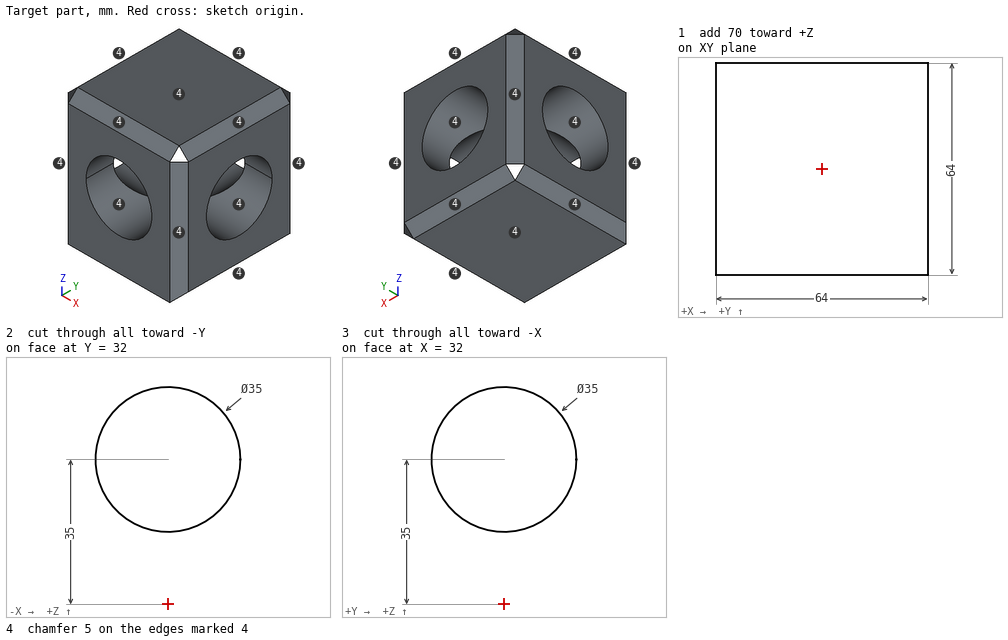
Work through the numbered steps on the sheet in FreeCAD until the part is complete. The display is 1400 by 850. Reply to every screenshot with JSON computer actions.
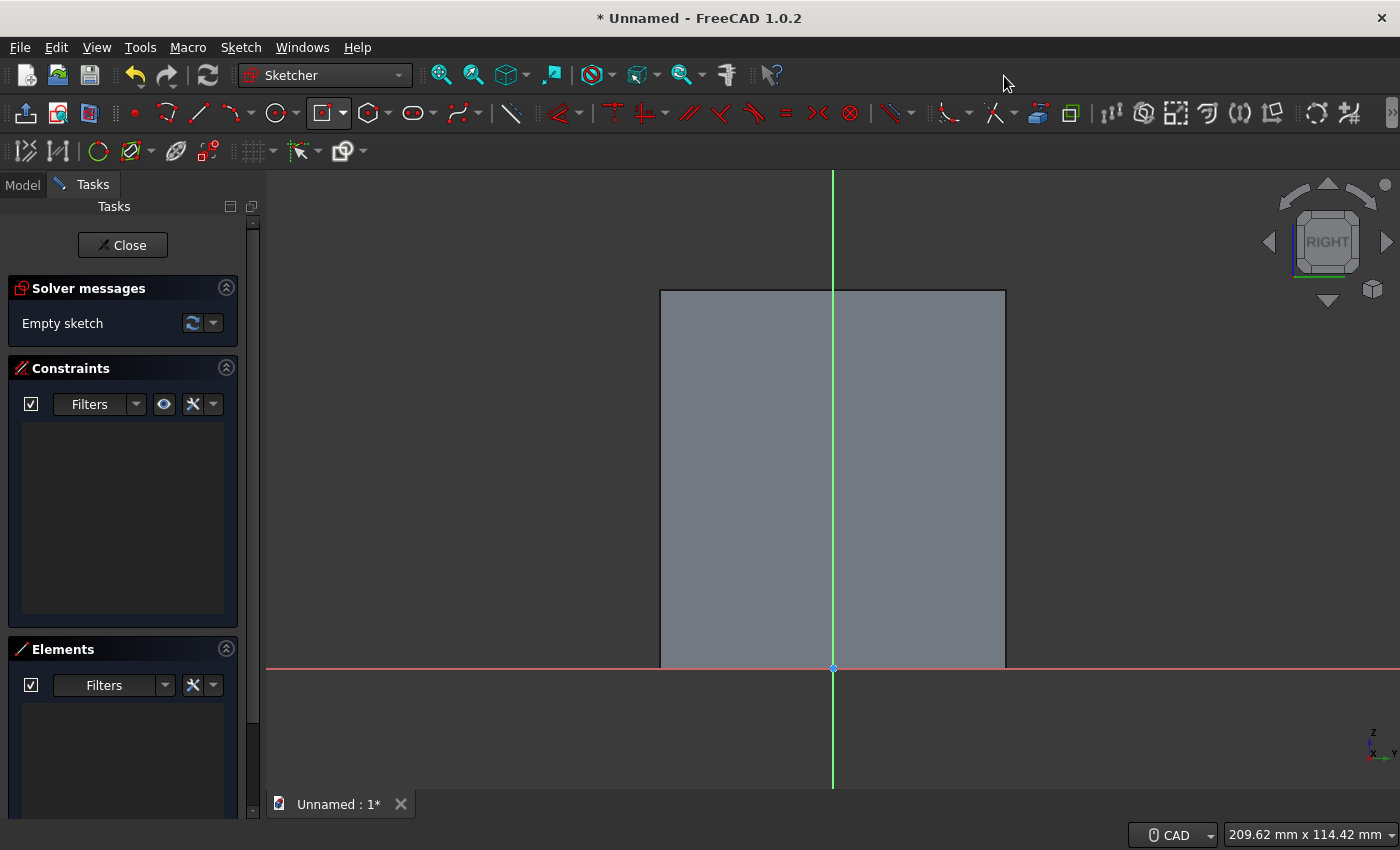
{"action": "scroll", "coordinate": [972, 623], "scroll_direction": "up", "scroll_amount": 2}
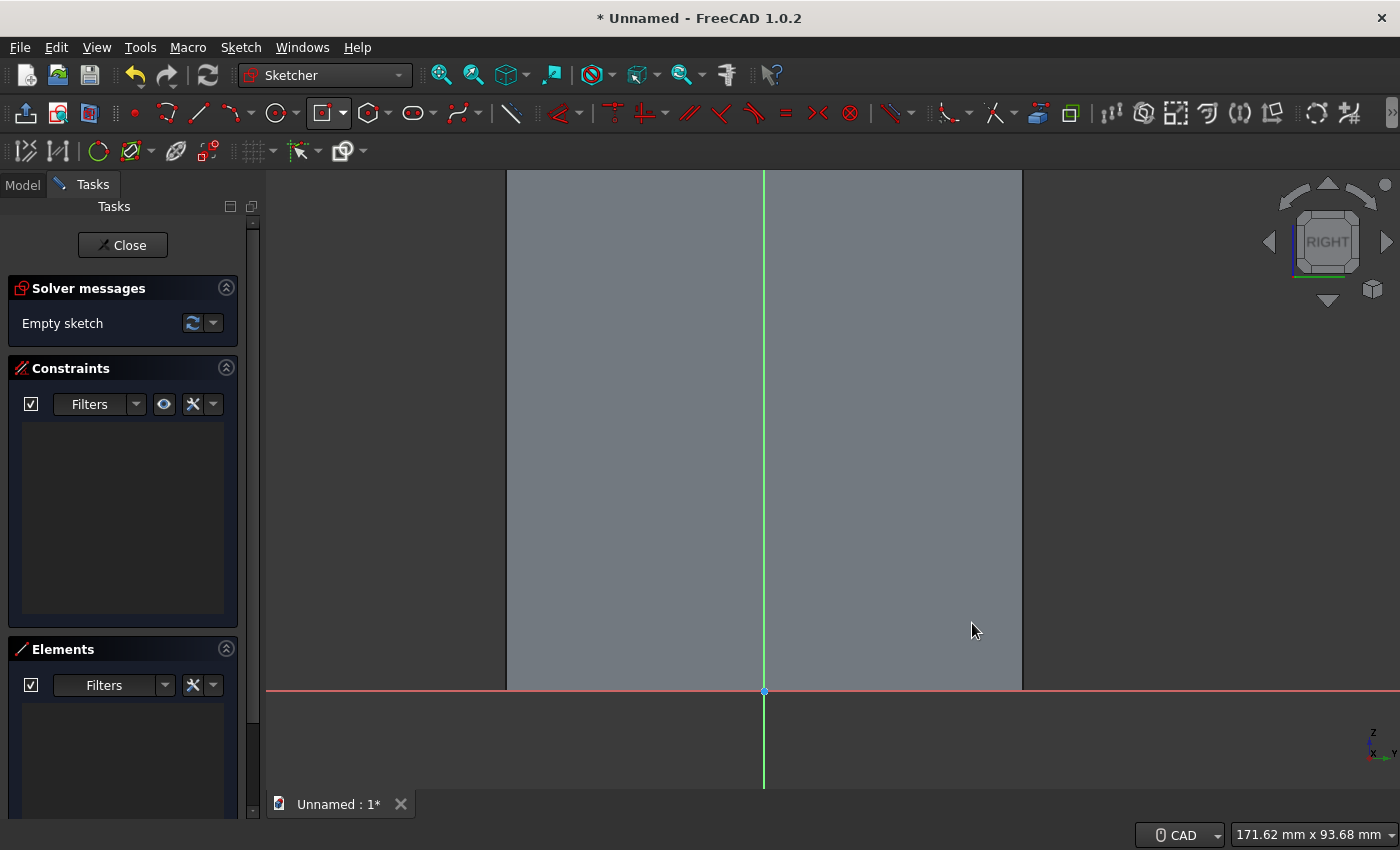
{"action": "key", "text": "g c"}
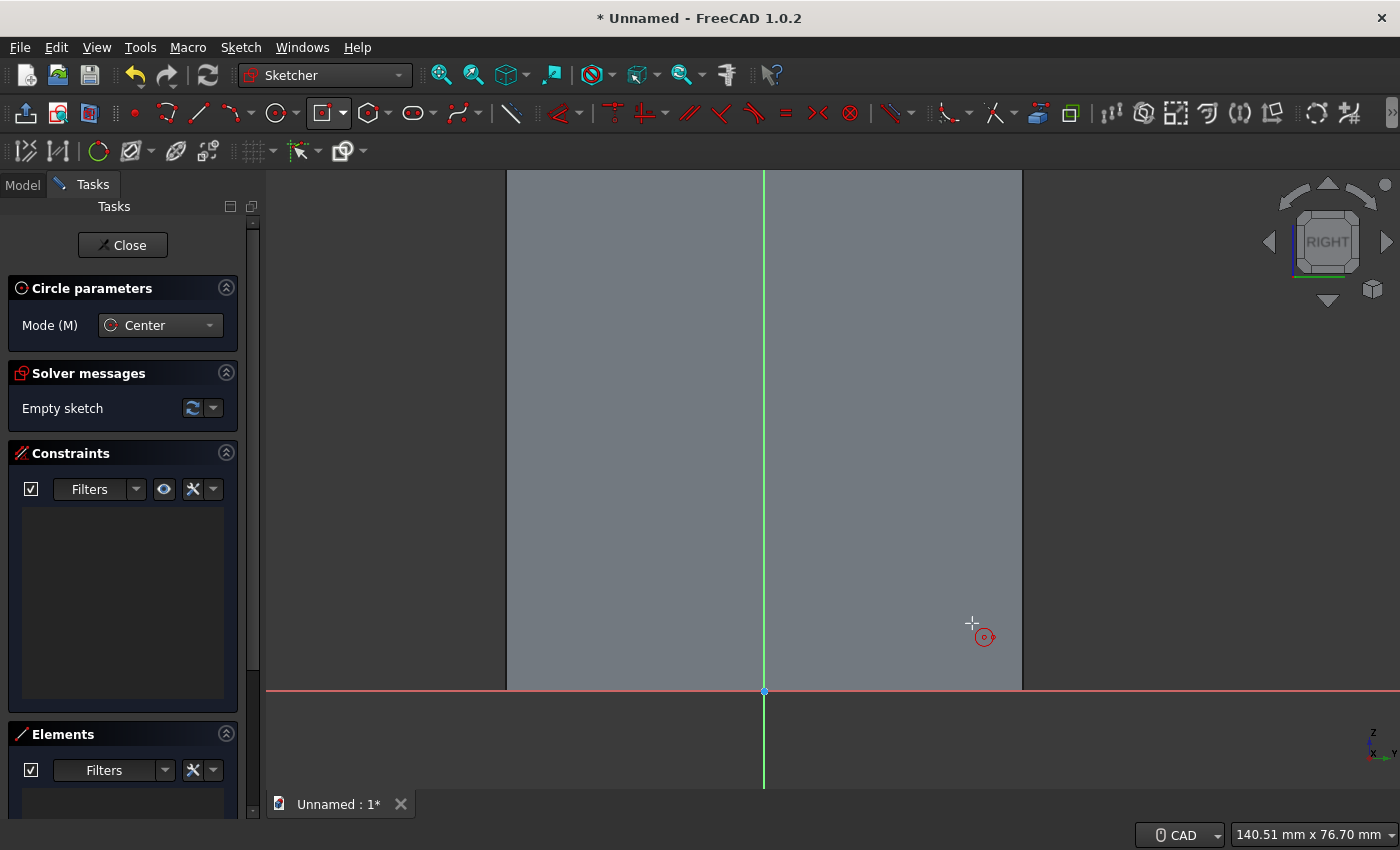
{"action": "left_click", "coordinate": [764, 409]}
{"action": "left_click", "coordinate": [864, 309]}
{"action": "key", "text": "Escape"}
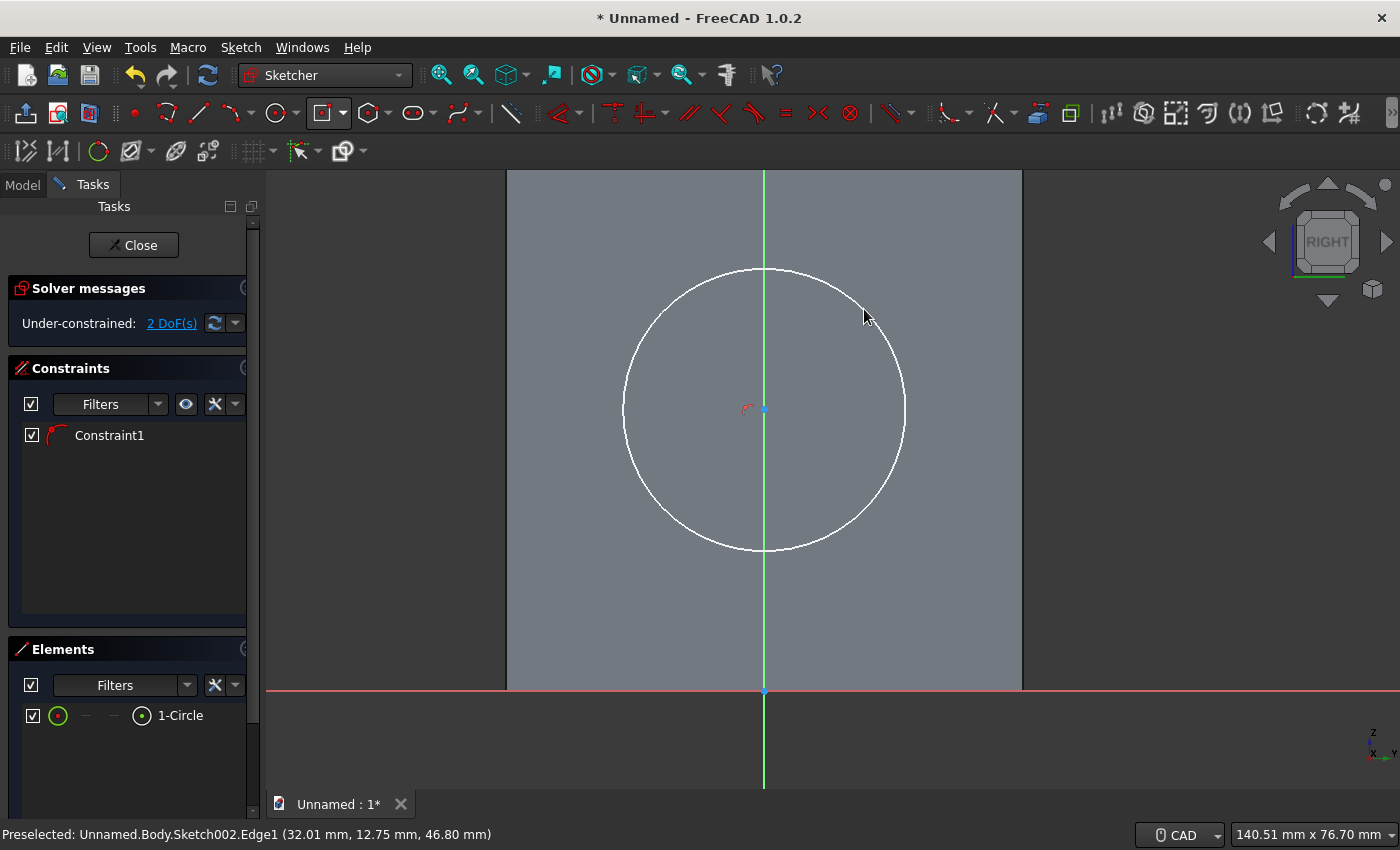
{"action": "left_click", "coordinate": [558, 114]}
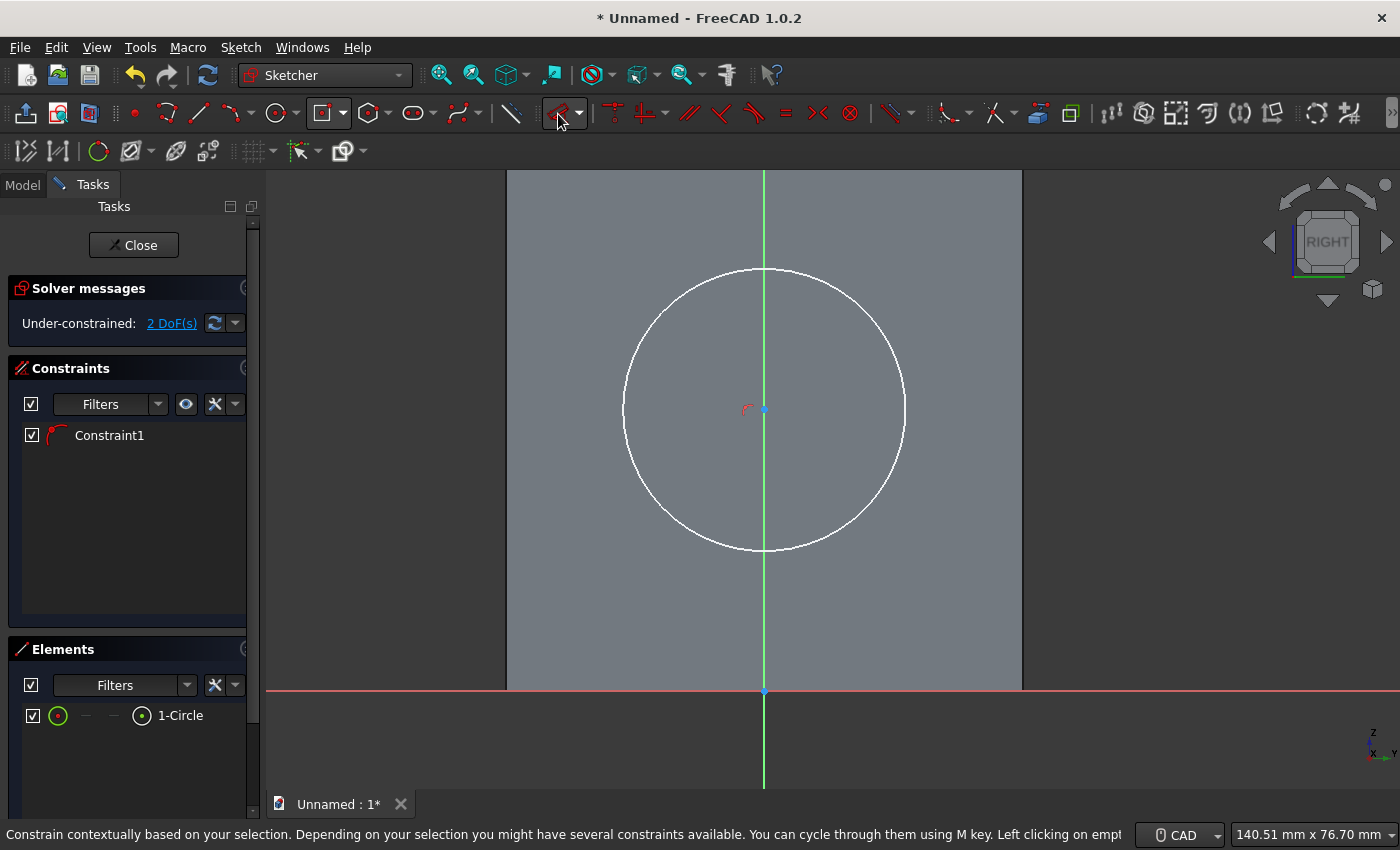
{"action": "left_click", "coordinate": [864, 310]}
{"action": "left_click", "coordinate": [887, 287]}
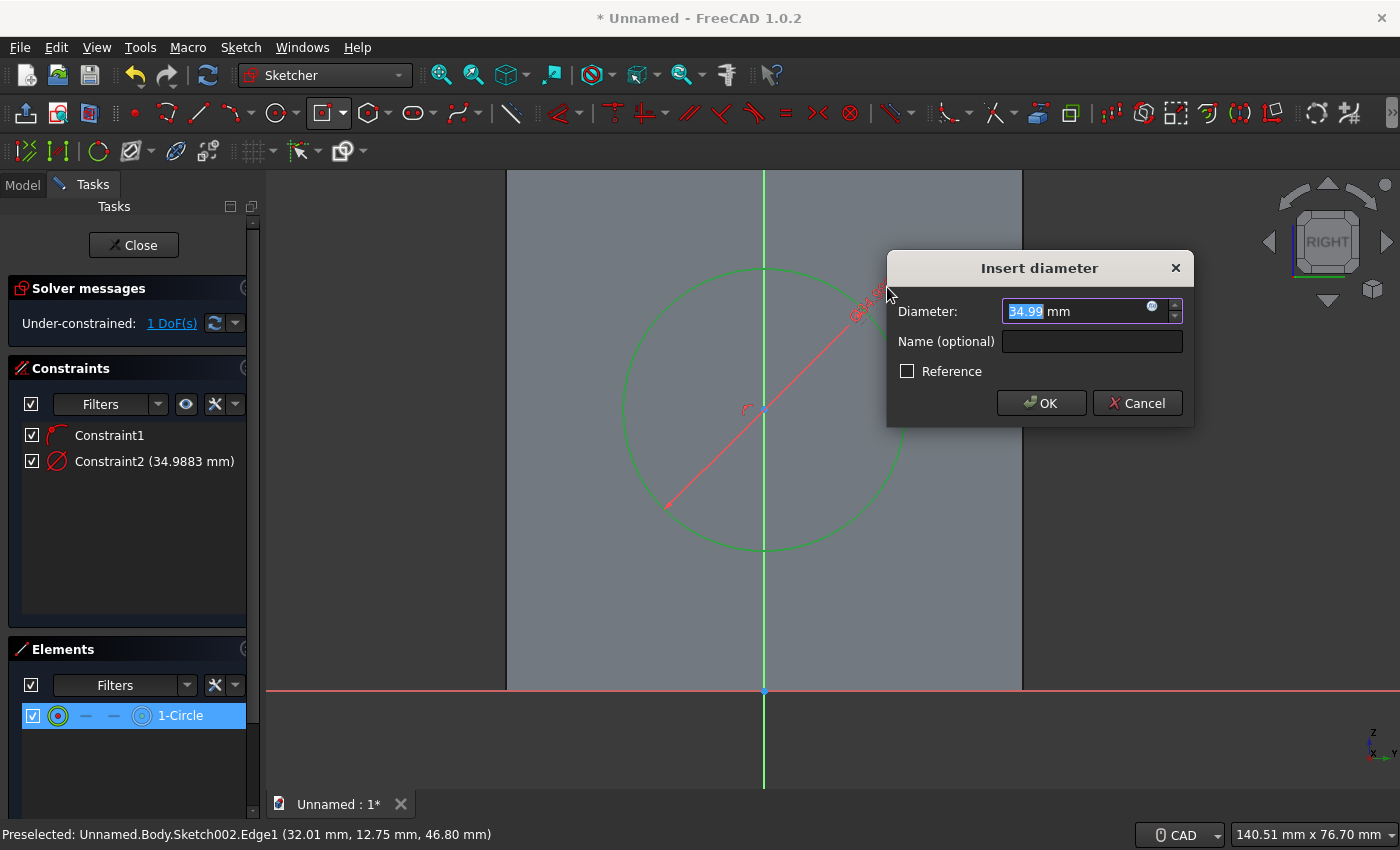
{"action": "type", "text": "35"}
{"action": "key", "text": "Return"}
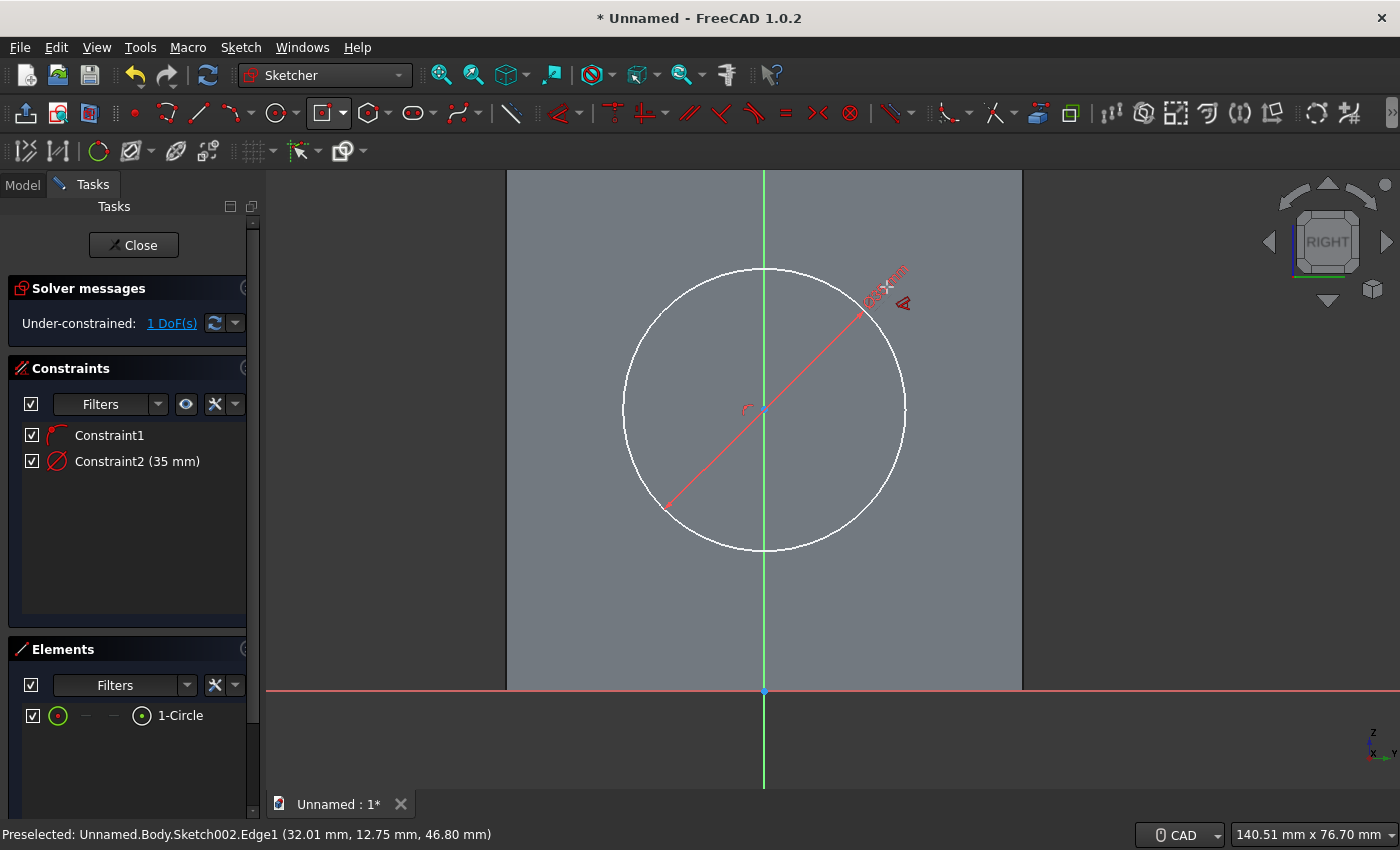
{"action": "left_click", "coordinate": [764, 410]}
{"action": "left_click", "coordinate": [798, 486]}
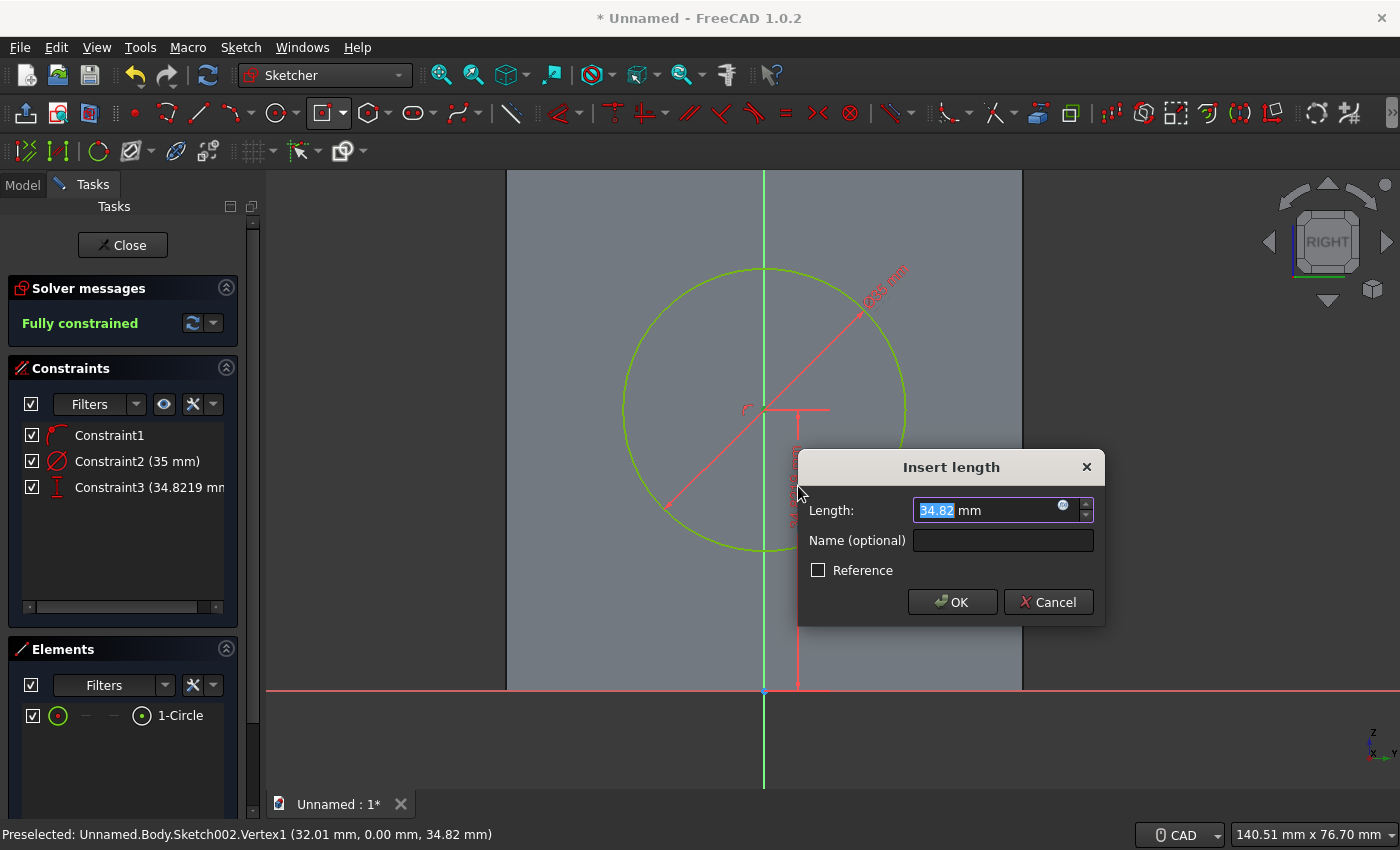
{"action": "type", "text": "35"}
{"action": "key", "text": "Return"}
{"action": "key", "text": "Escape"}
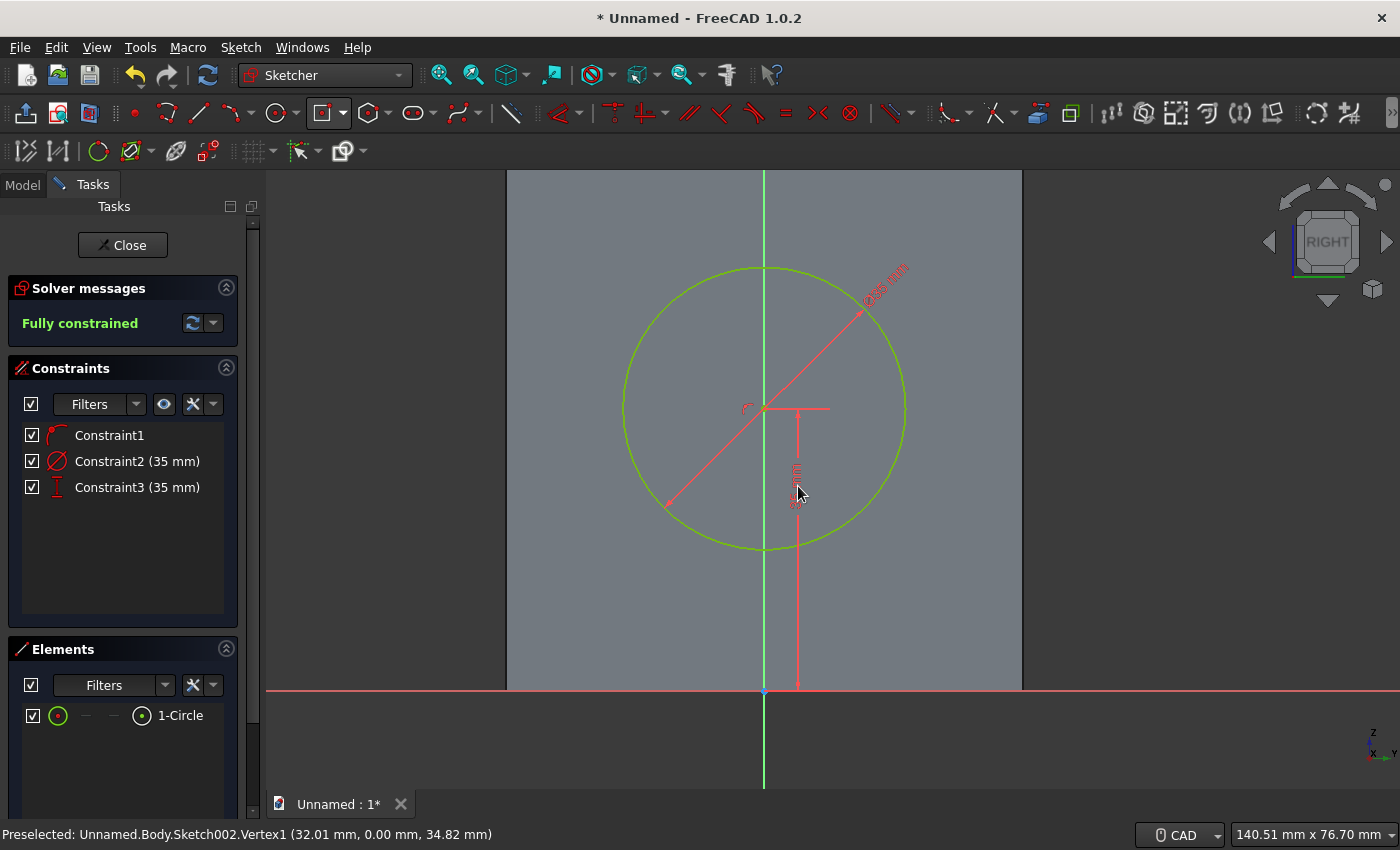
{"action": "left_click", "coordinate": [123, 245]}